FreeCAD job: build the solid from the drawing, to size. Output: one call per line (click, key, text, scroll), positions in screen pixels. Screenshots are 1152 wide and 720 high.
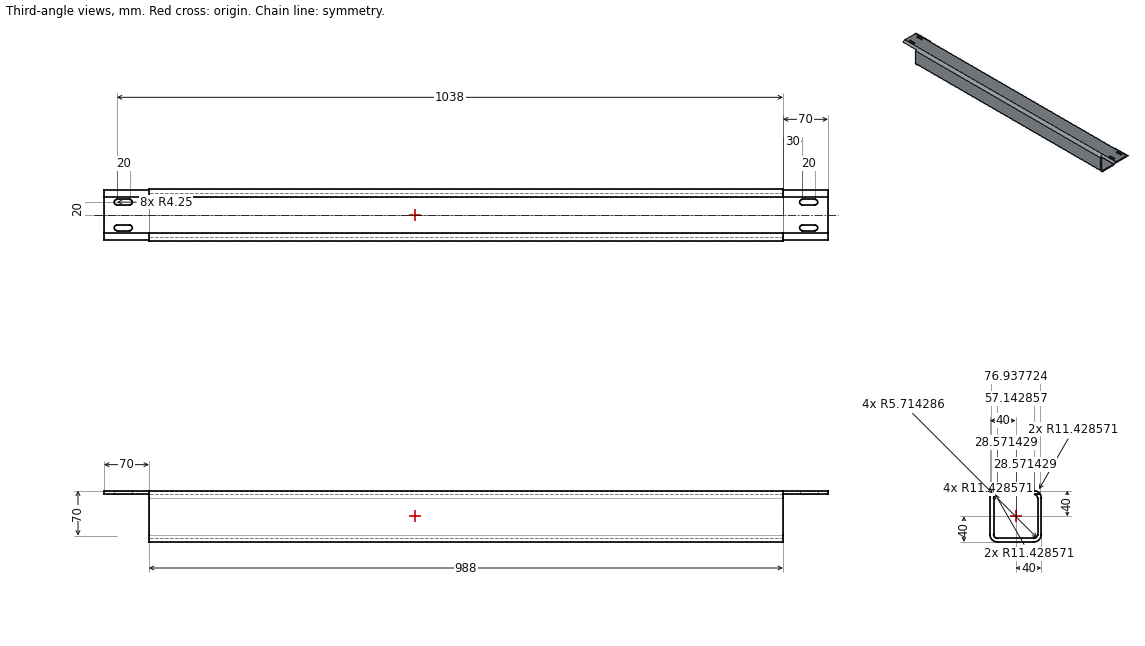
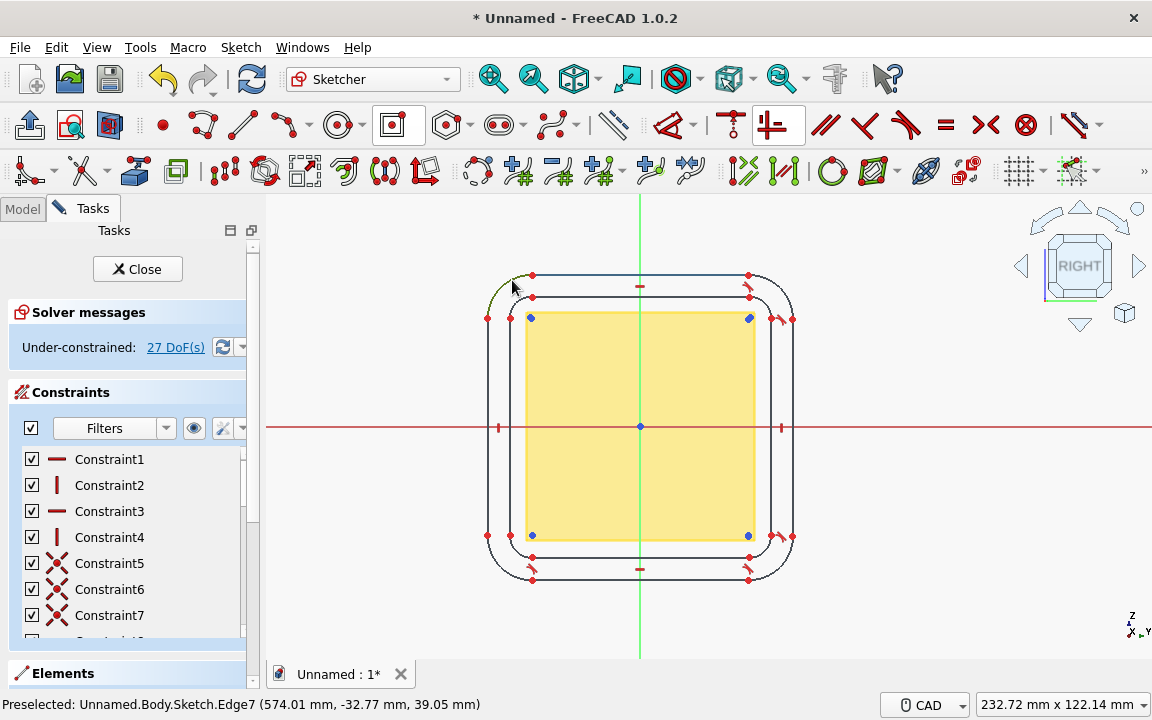
key(t)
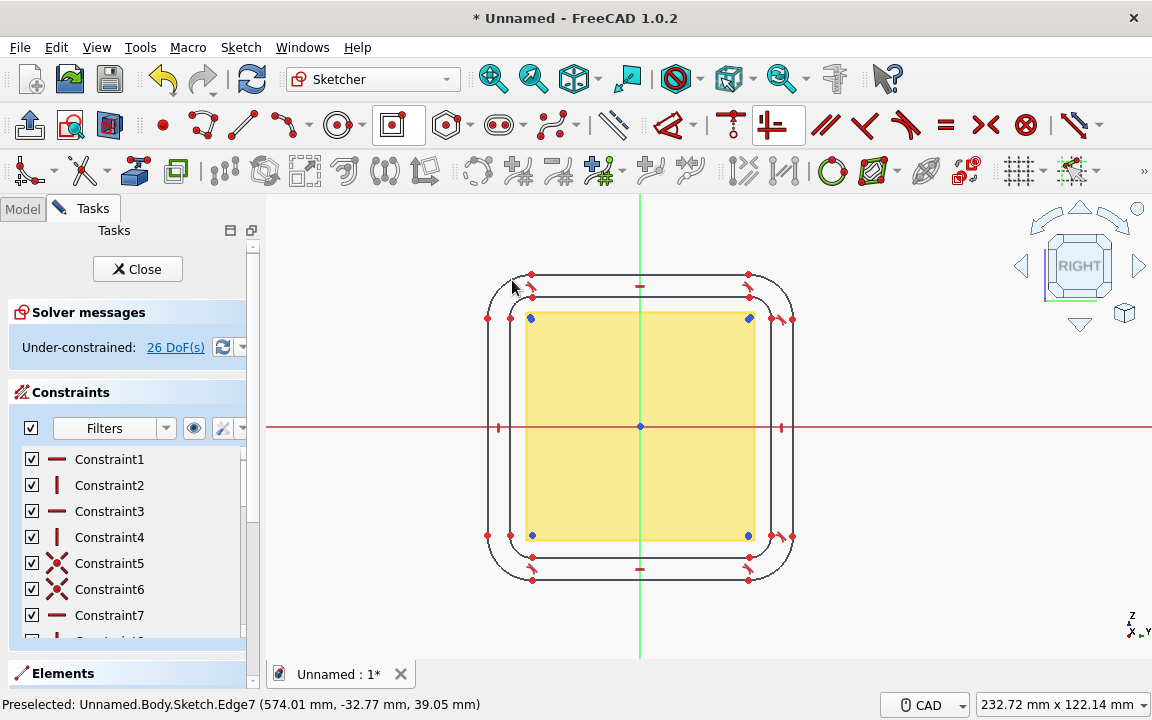
click(488, 384)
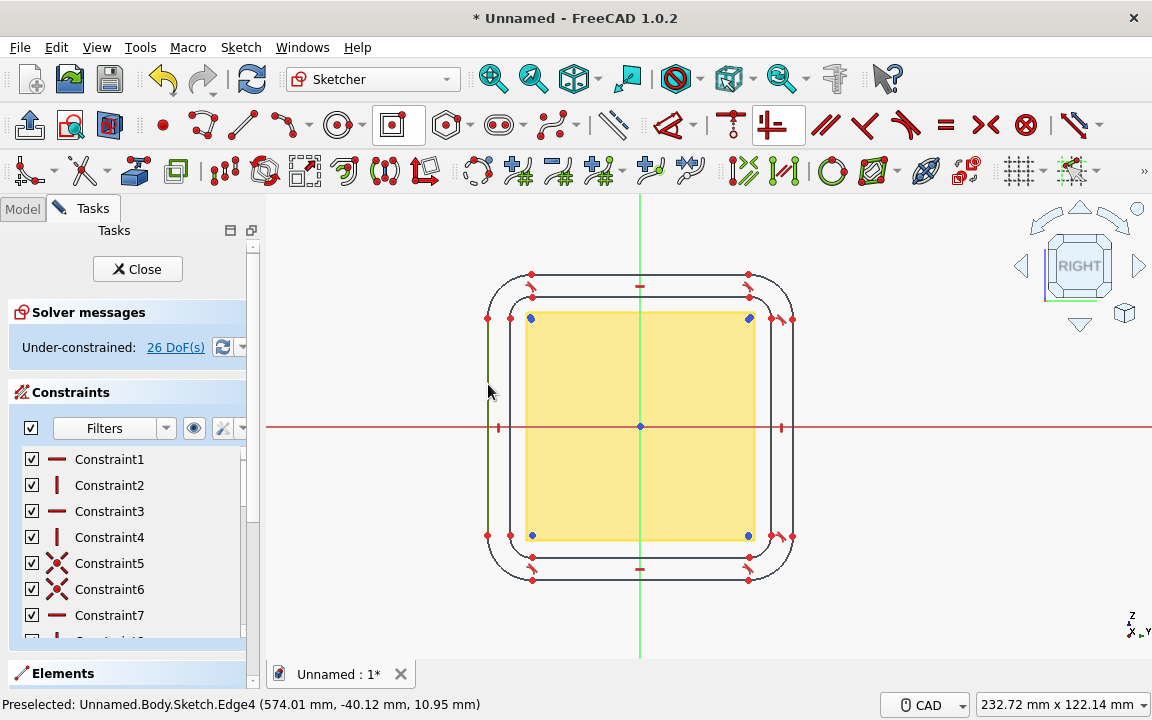
click(512, 280)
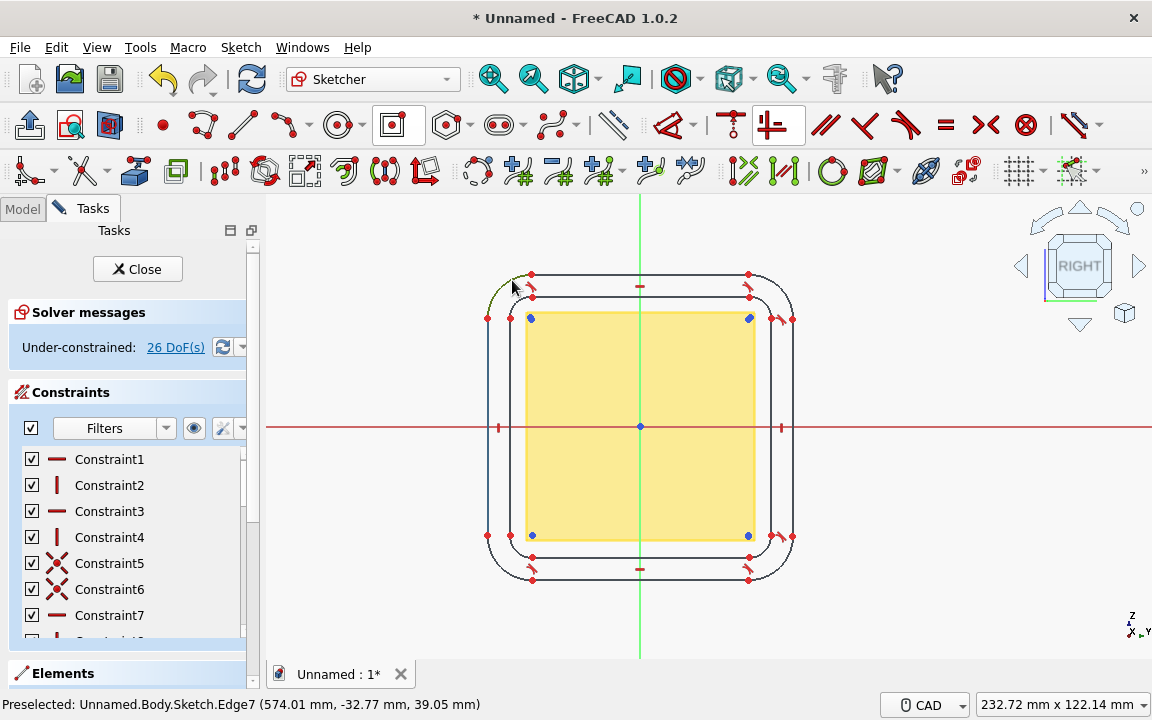
key(t)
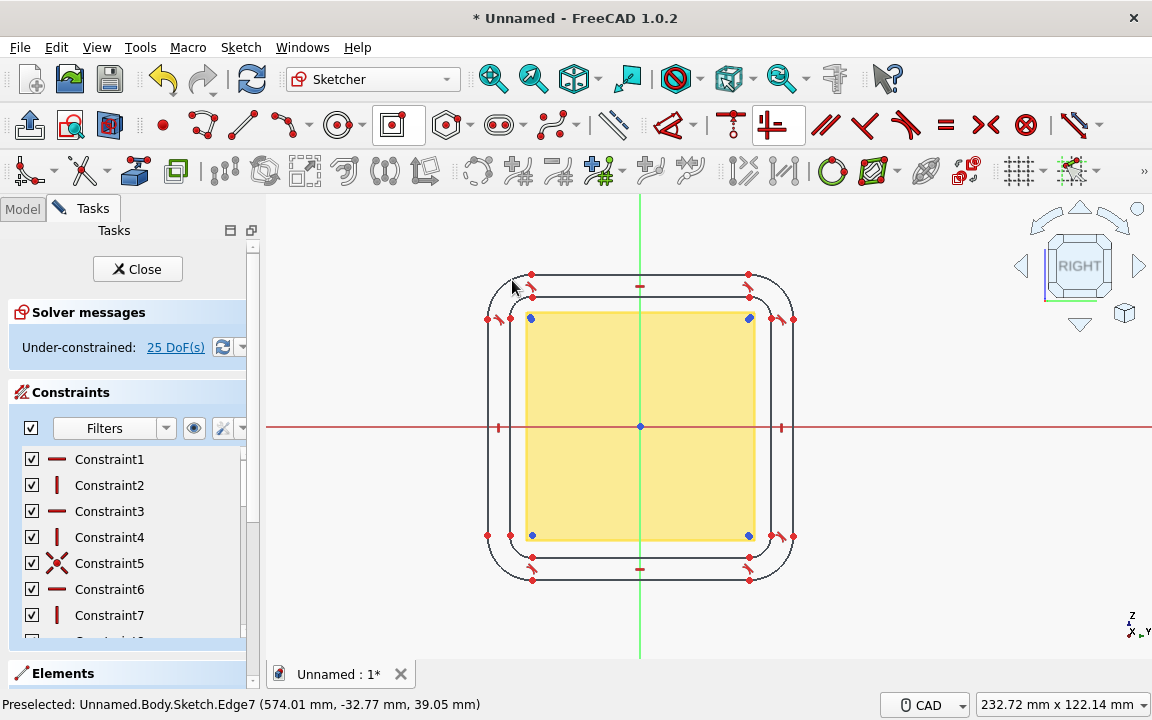
click(488, 384)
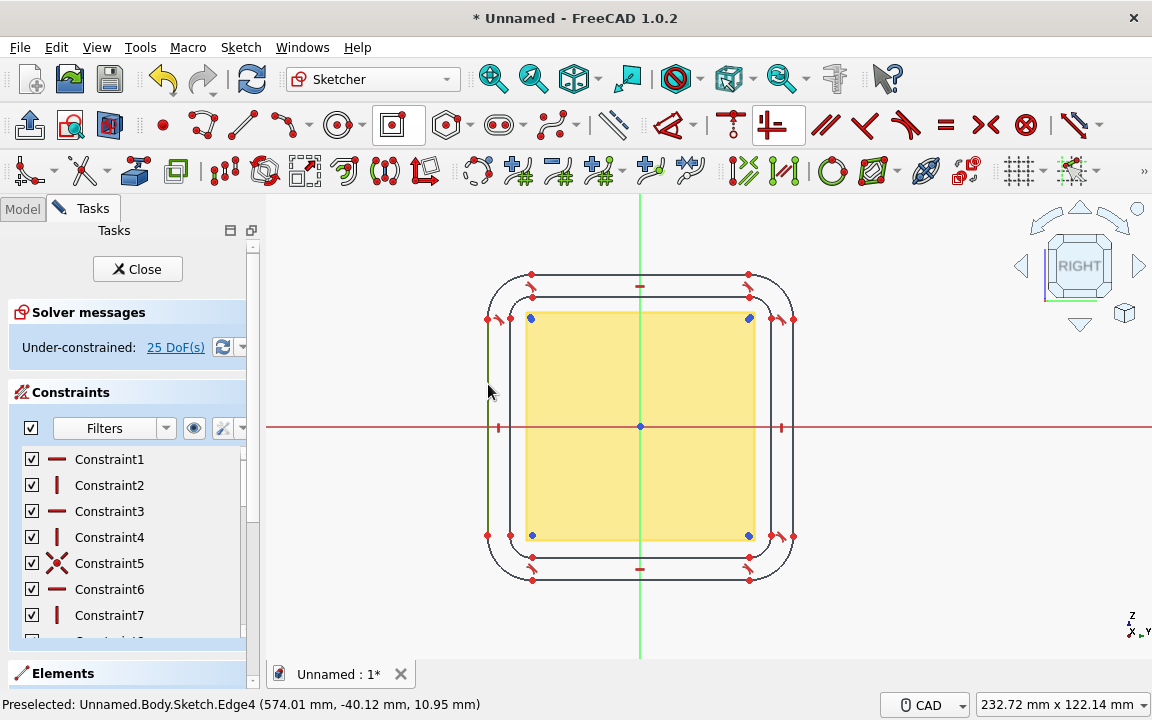
click(493, 556)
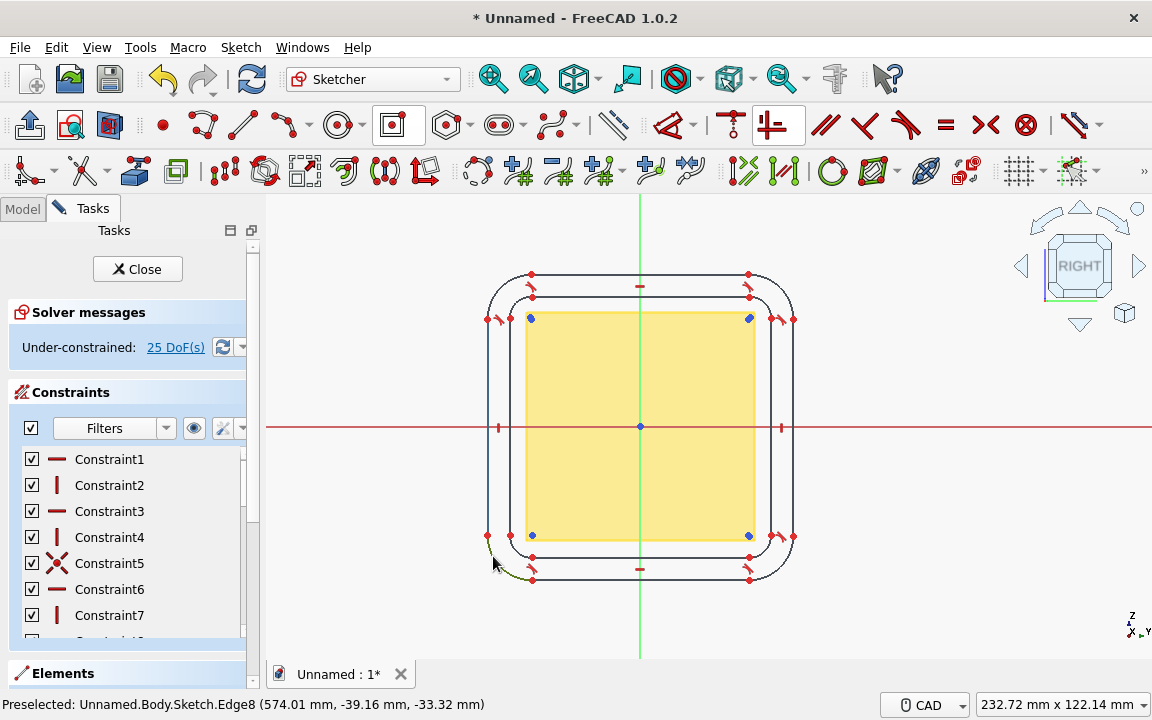
key(t)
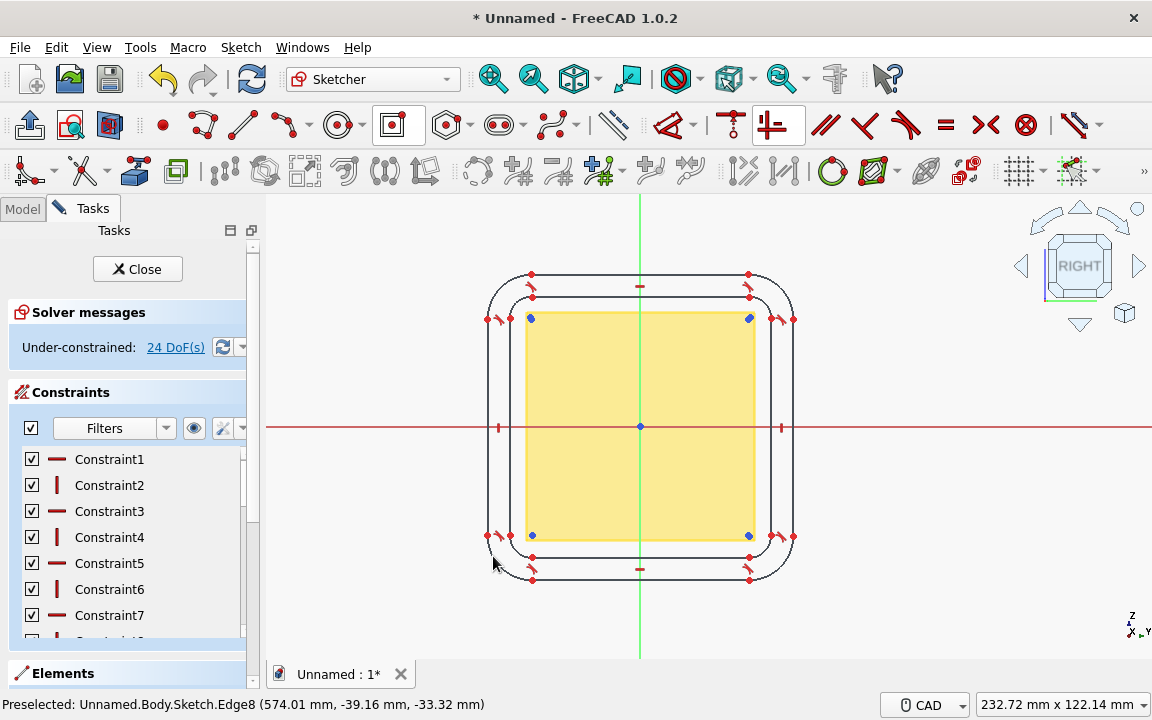
click(597, 297)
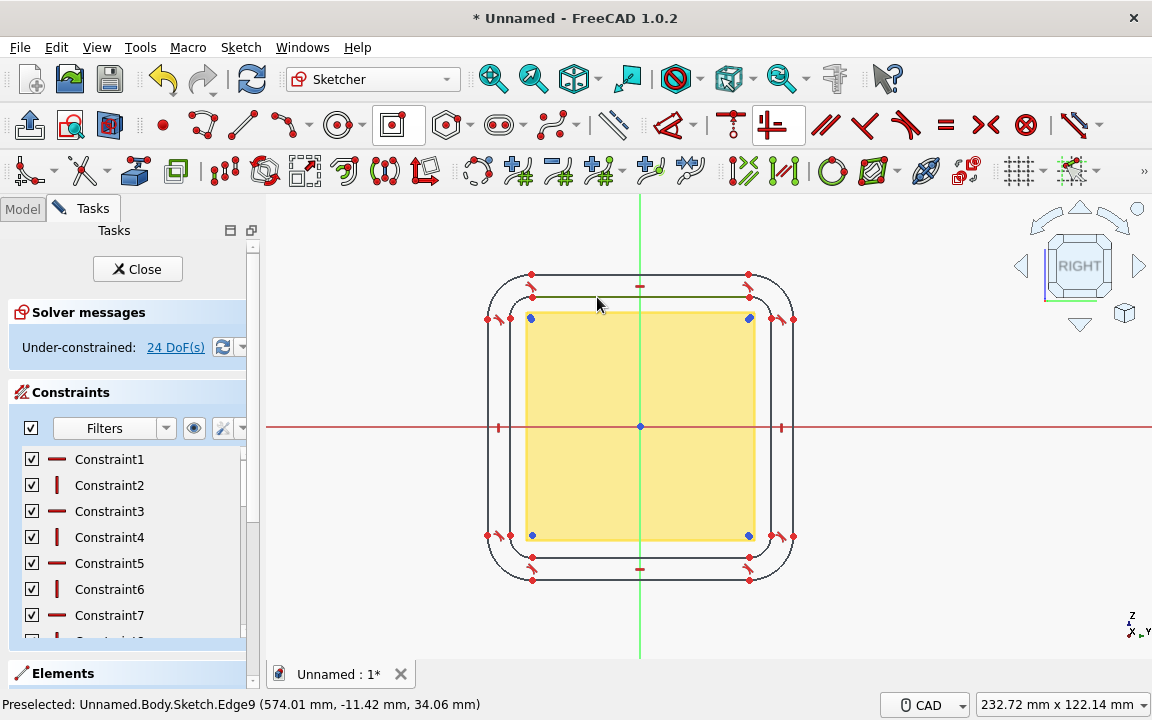
scroll(769, 309, up, 2)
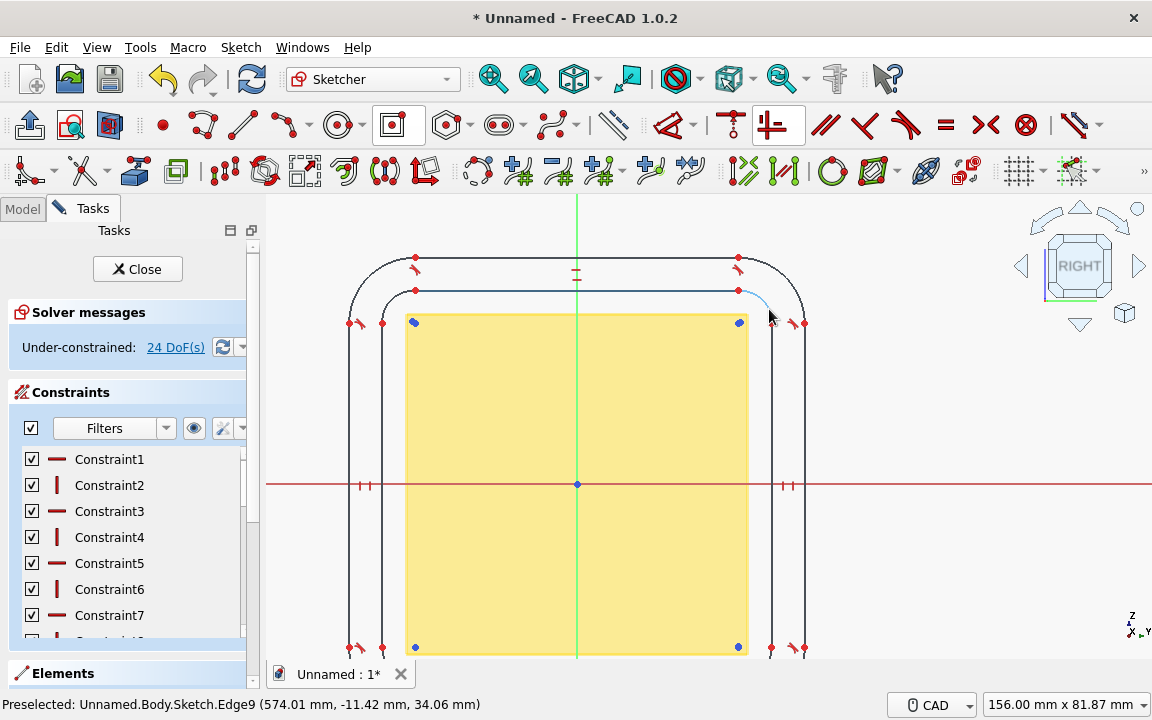
click(769, 309)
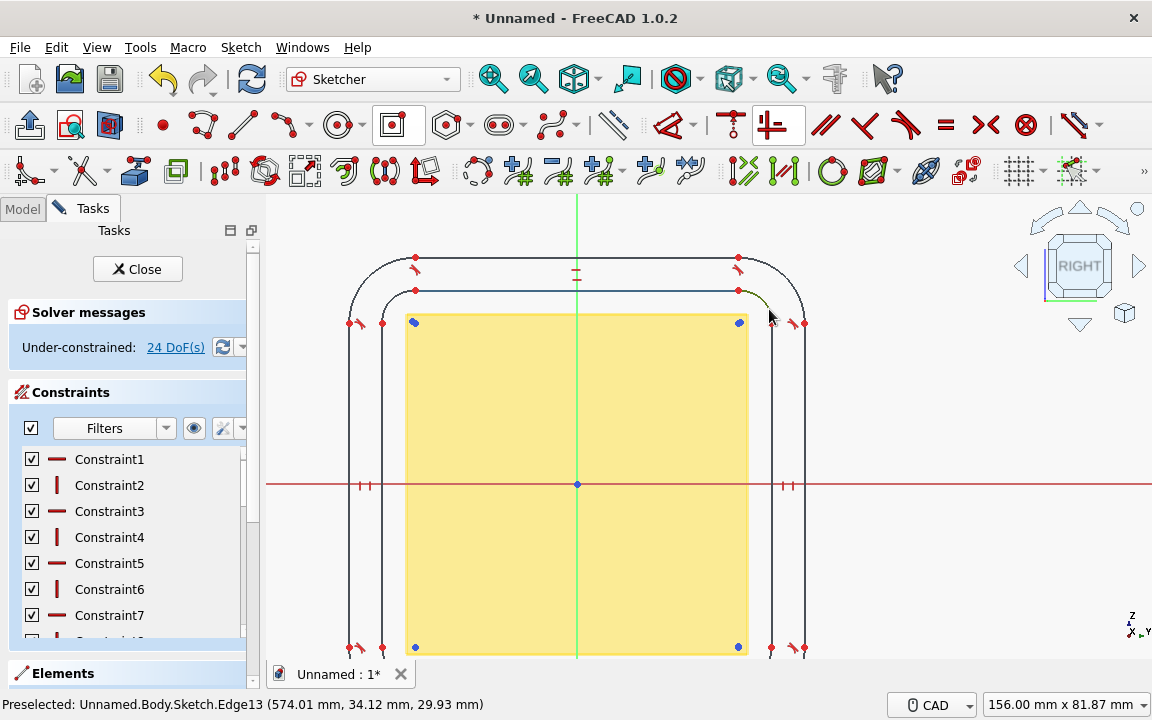
key(t)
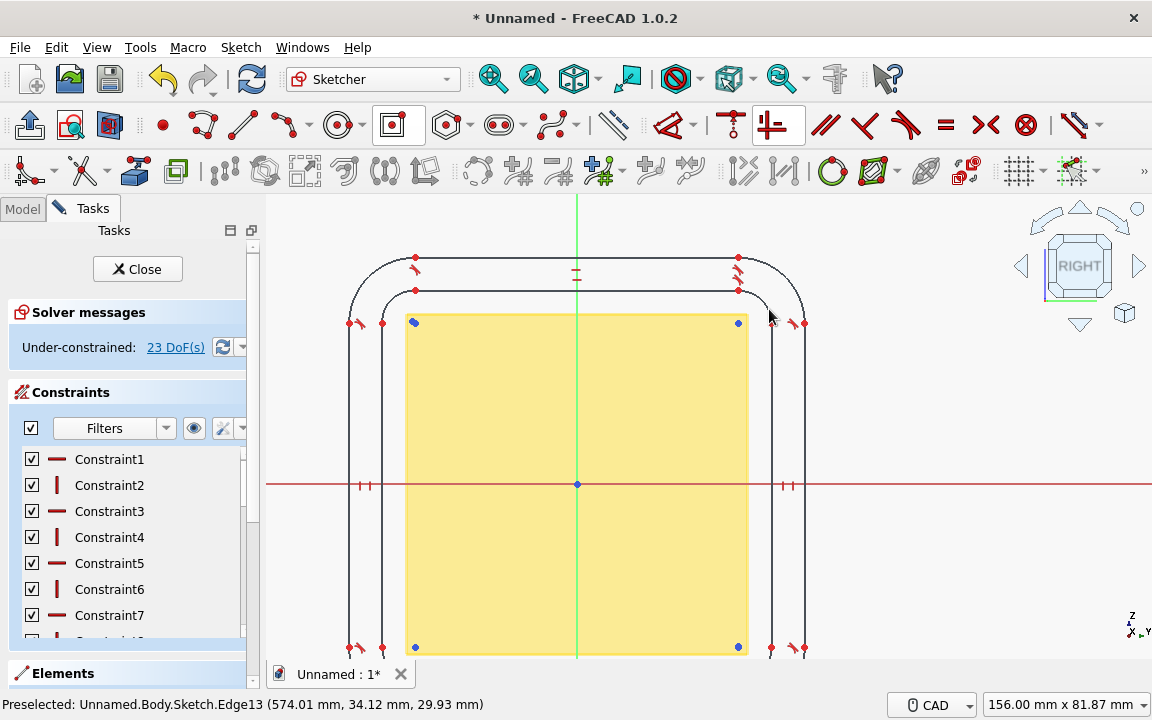
click(512, 291)